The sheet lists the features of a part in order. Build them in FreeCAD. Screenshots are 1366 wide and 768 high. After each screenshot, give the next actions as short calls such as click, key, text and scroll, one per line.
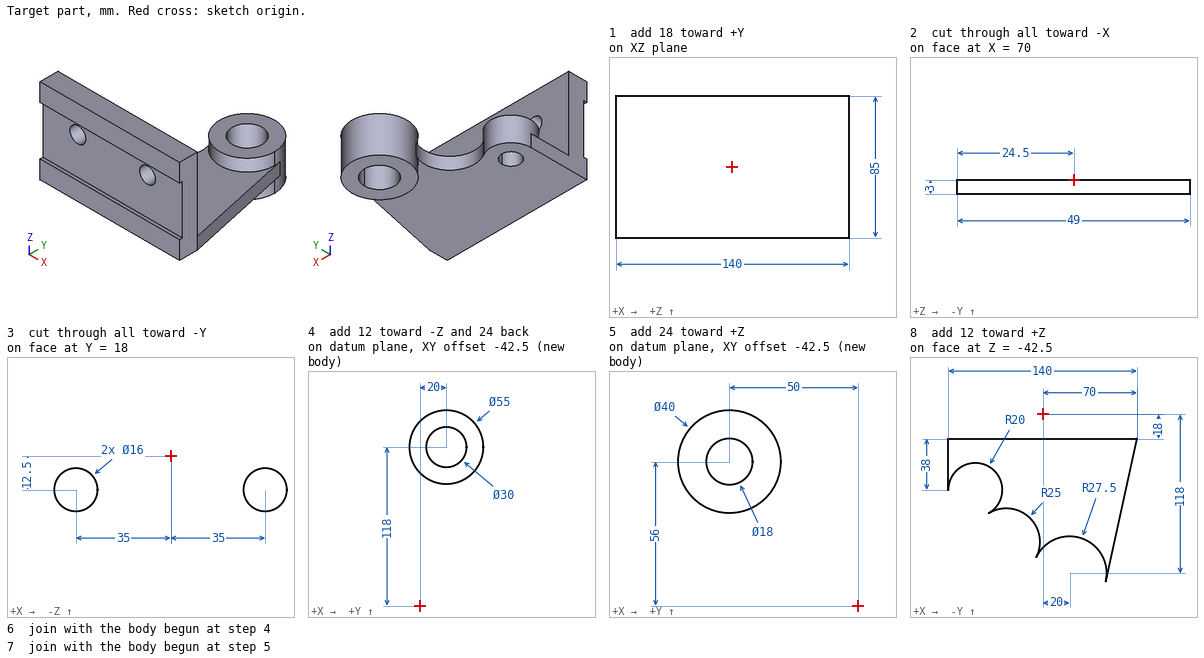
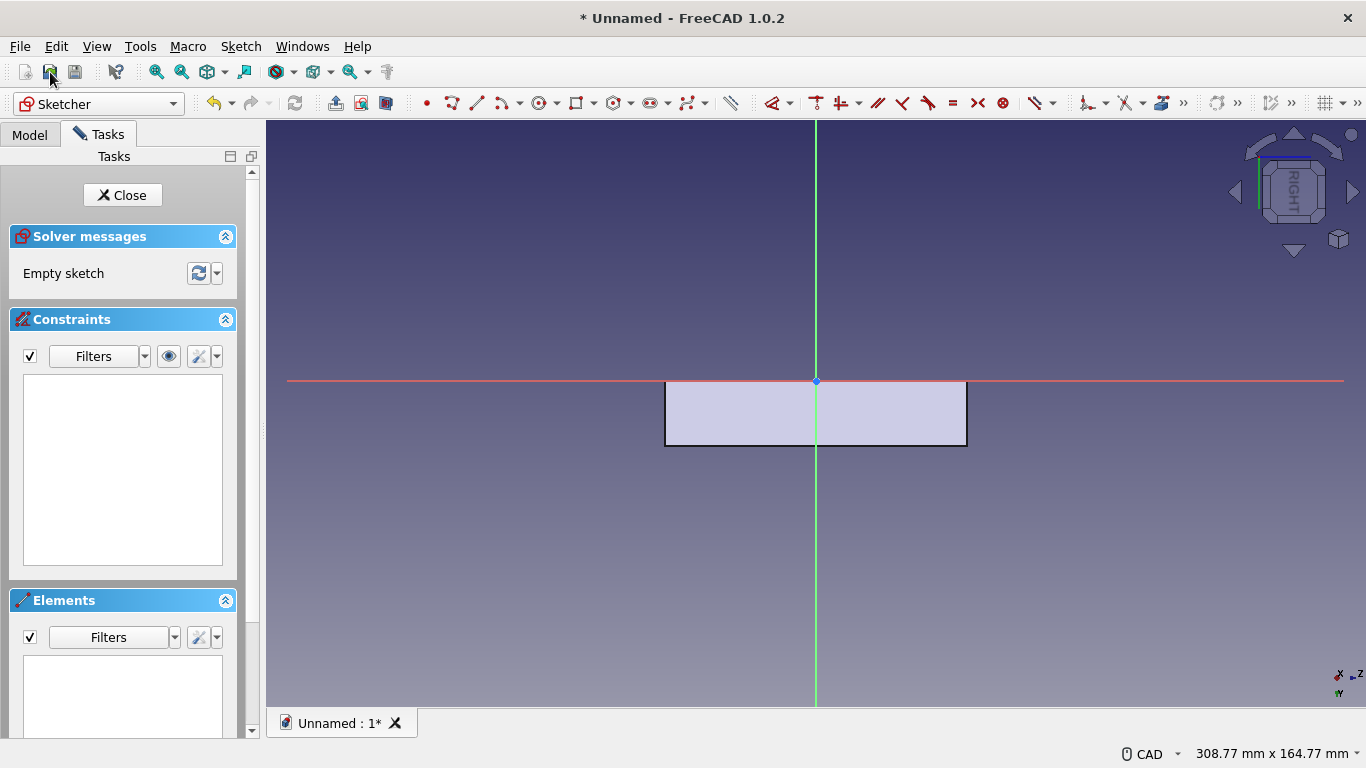
scroll(846, 375, up, 6)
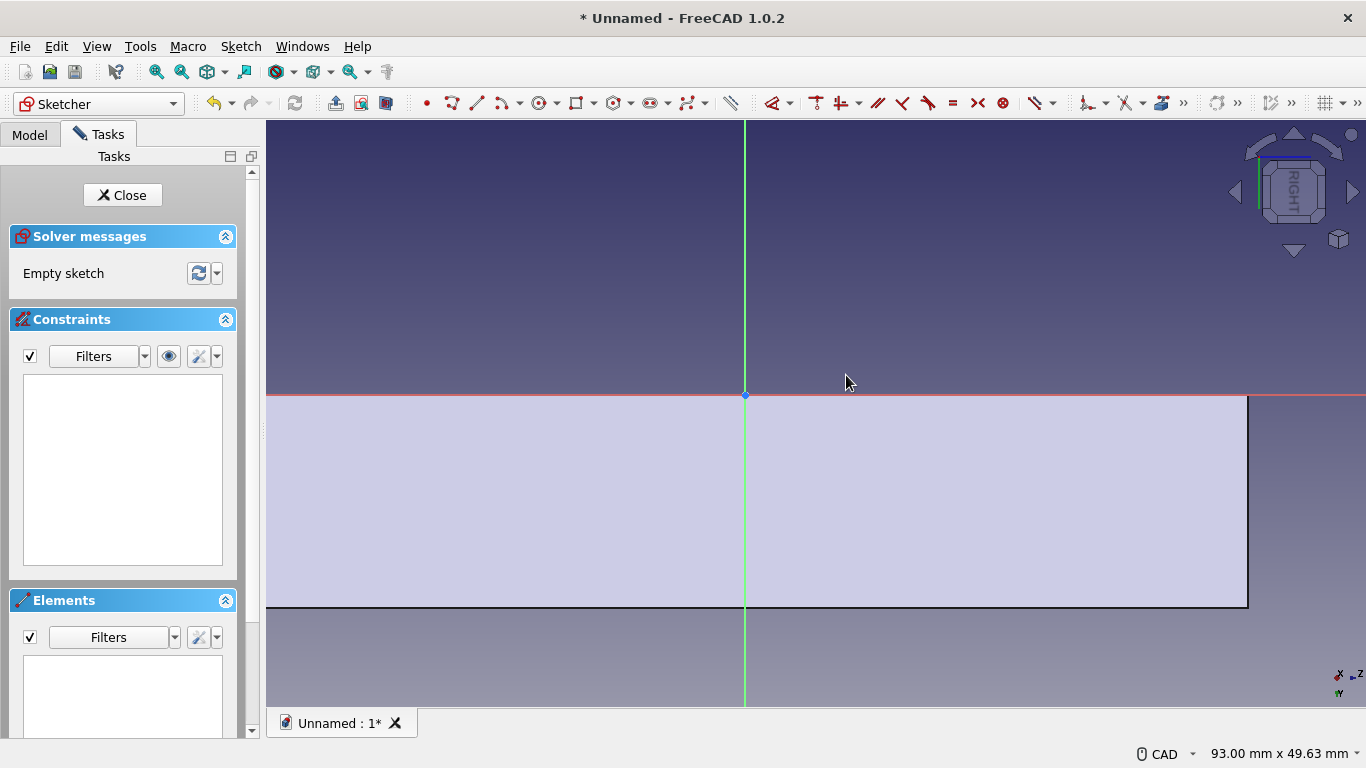
click(576, 104)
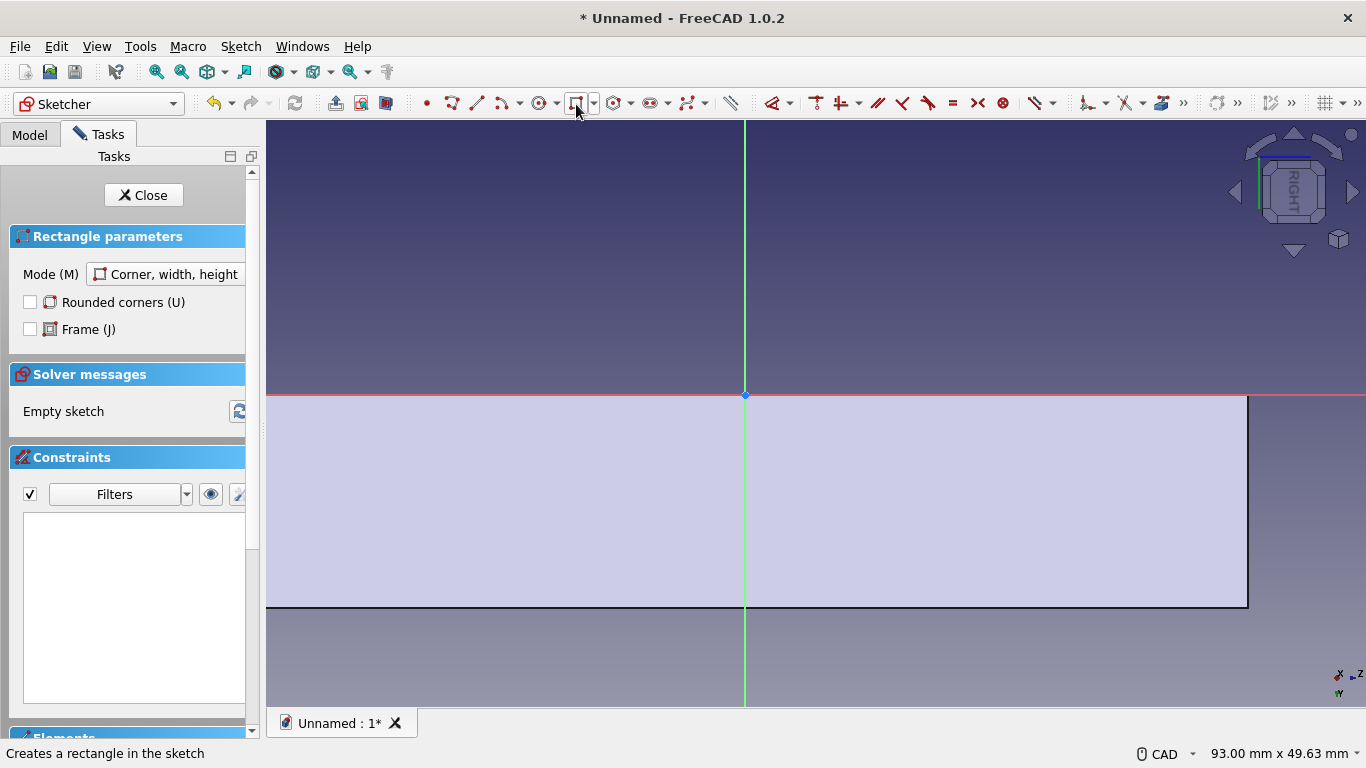
click(455, 395)
click(1035, 431)
key(Escape)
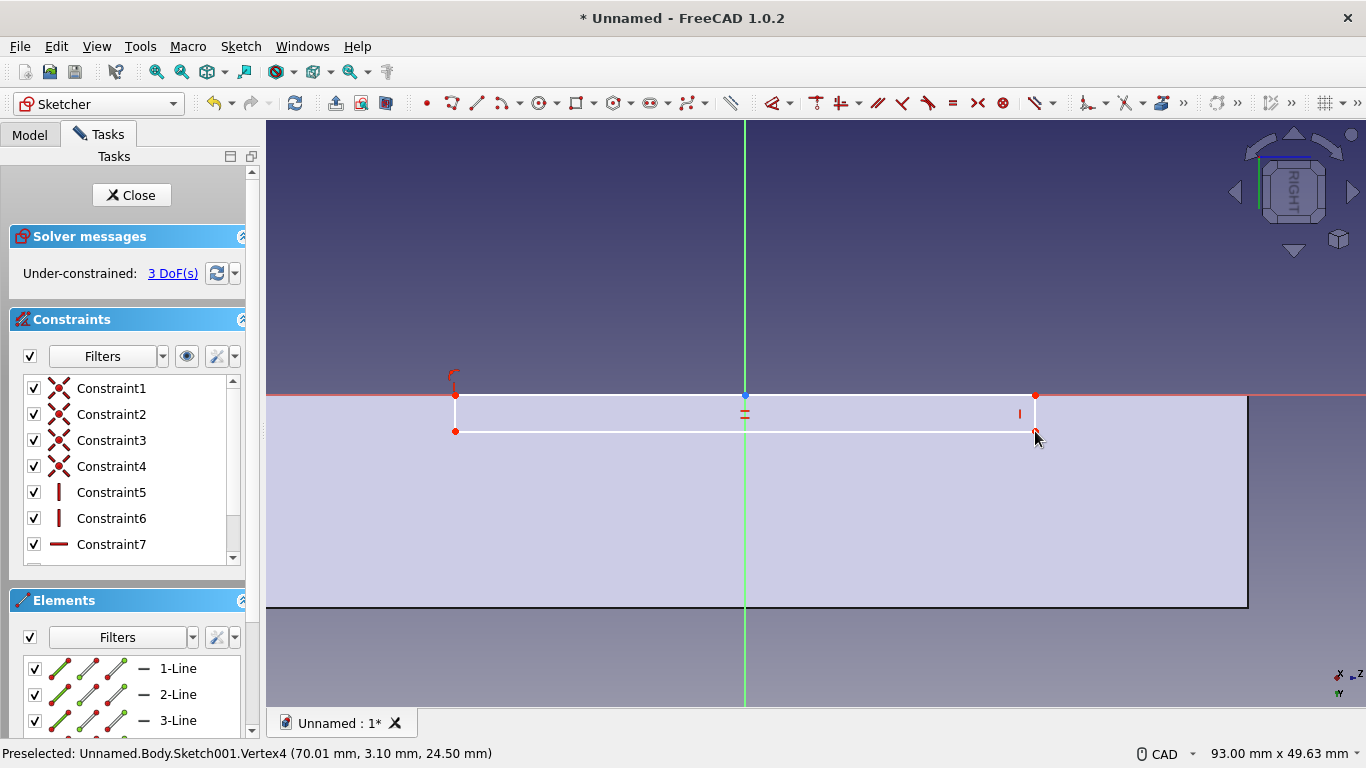
click(772, 104)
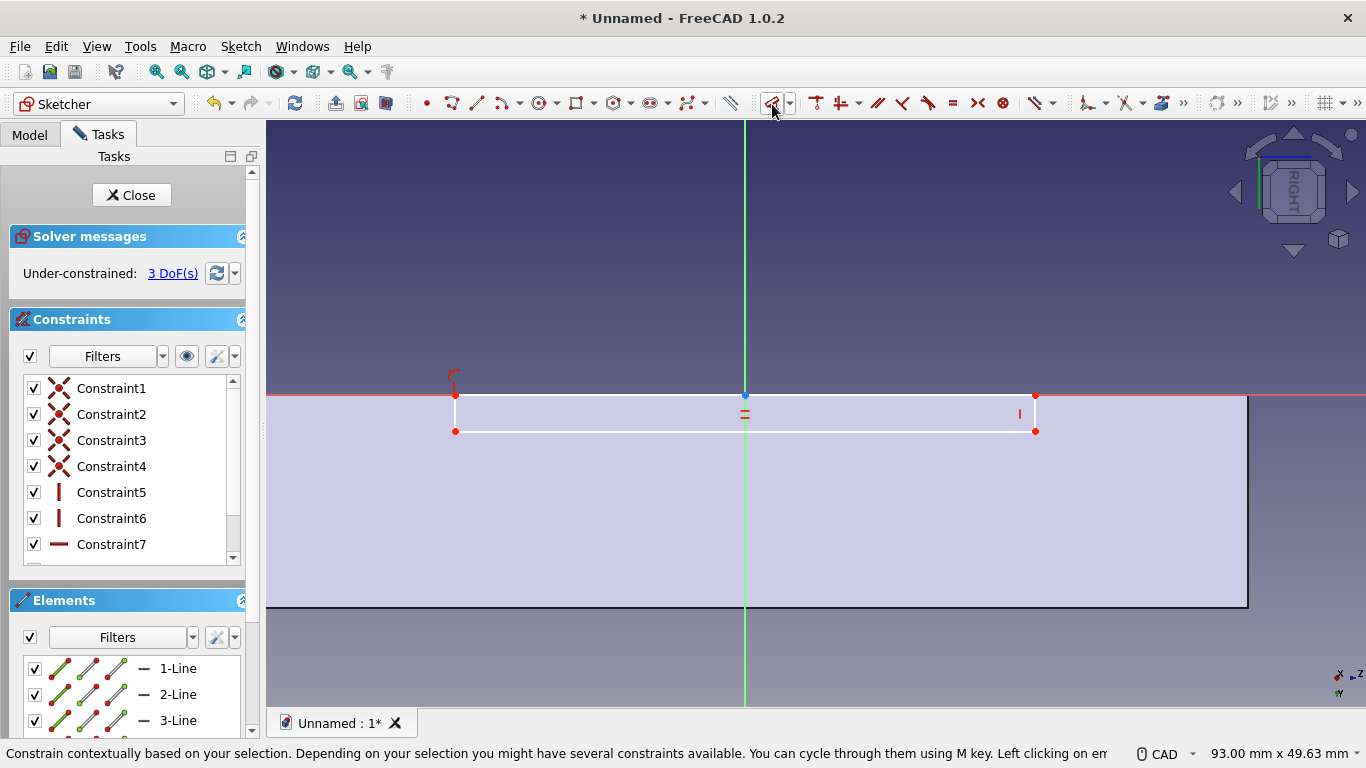
scroll(455, 406, up, 2)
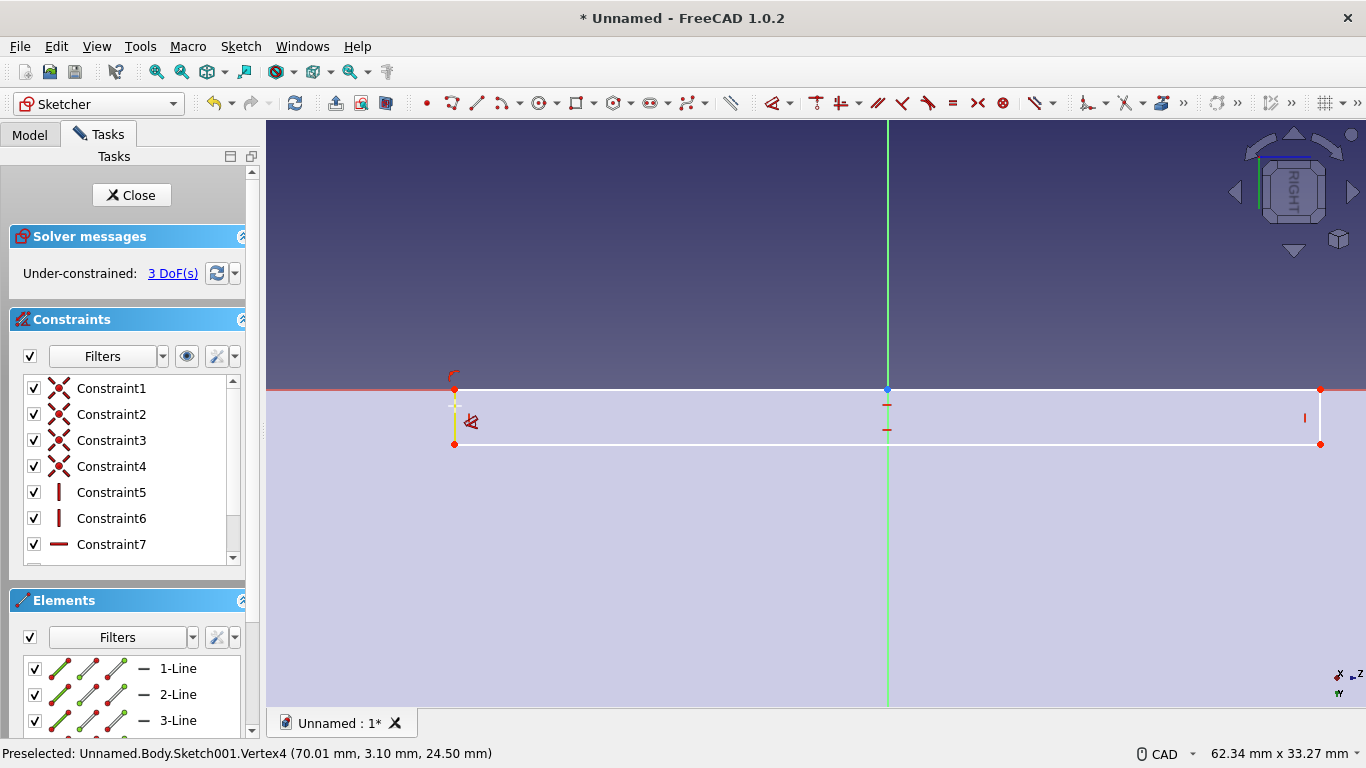
click(455, 406)
click(421, 417)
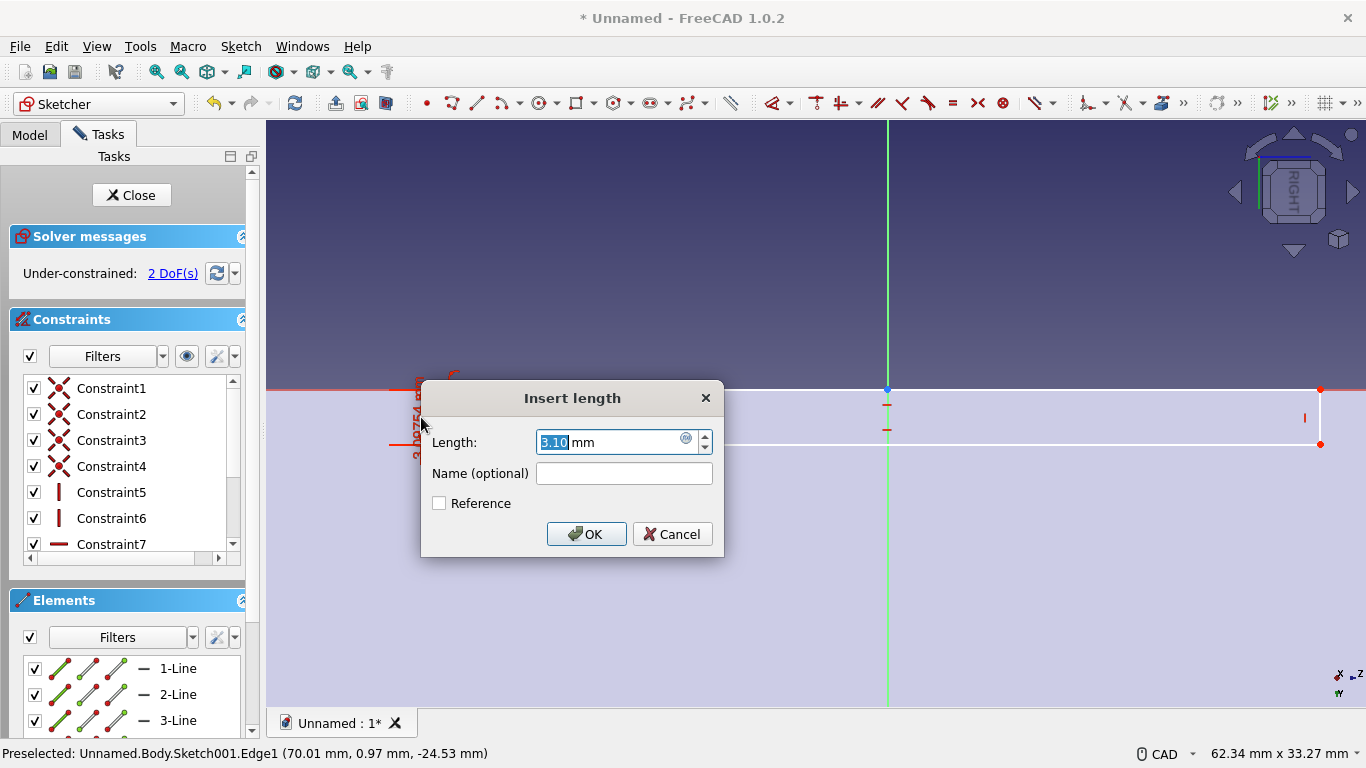
text(3)
key(Return)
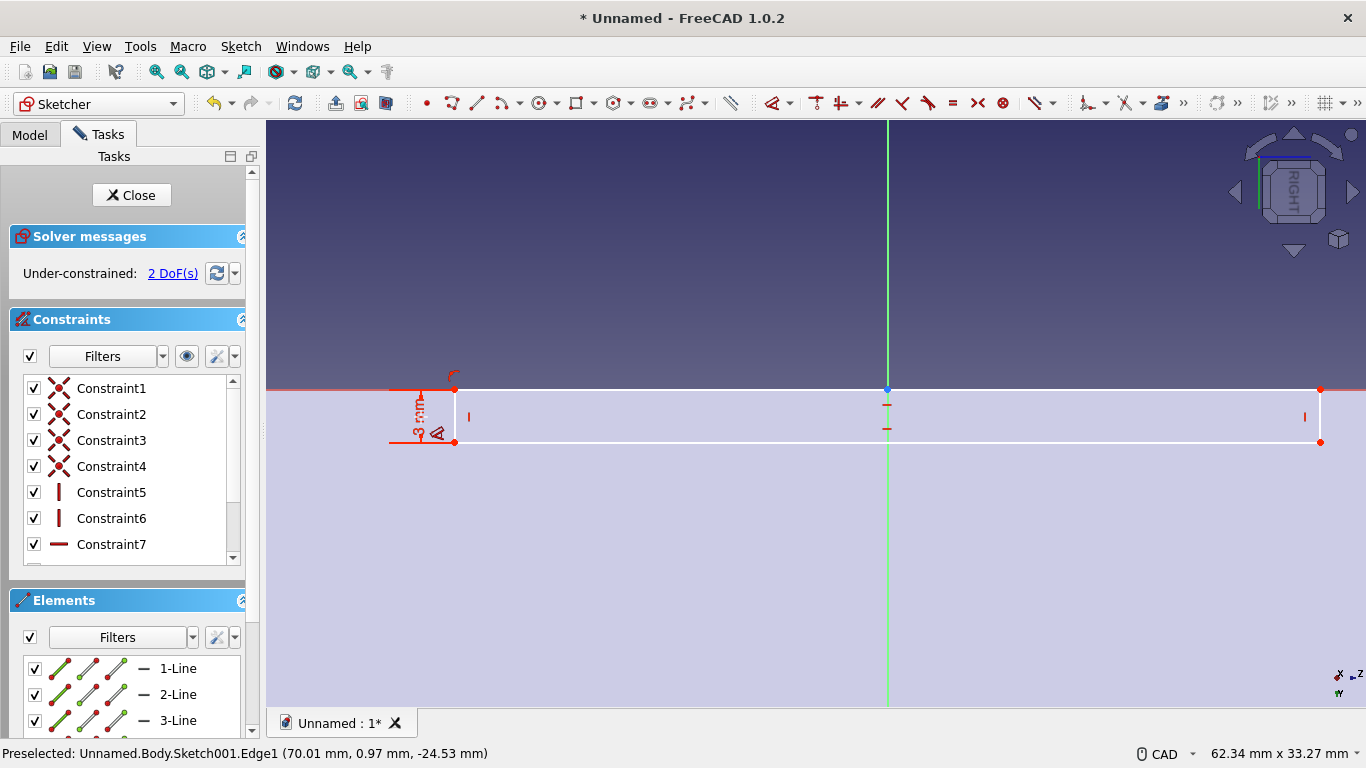
click(714, 443)
click(828, 477)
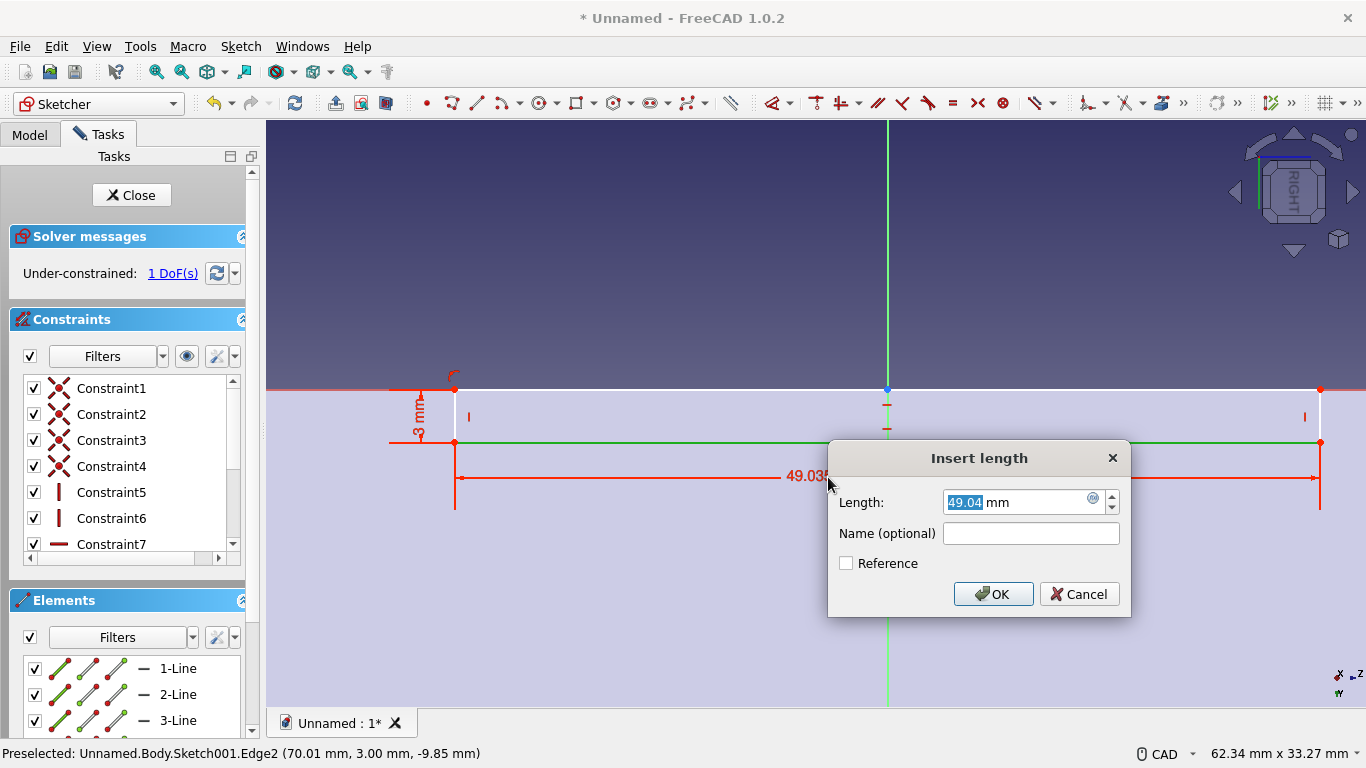
text(49)
key(Return)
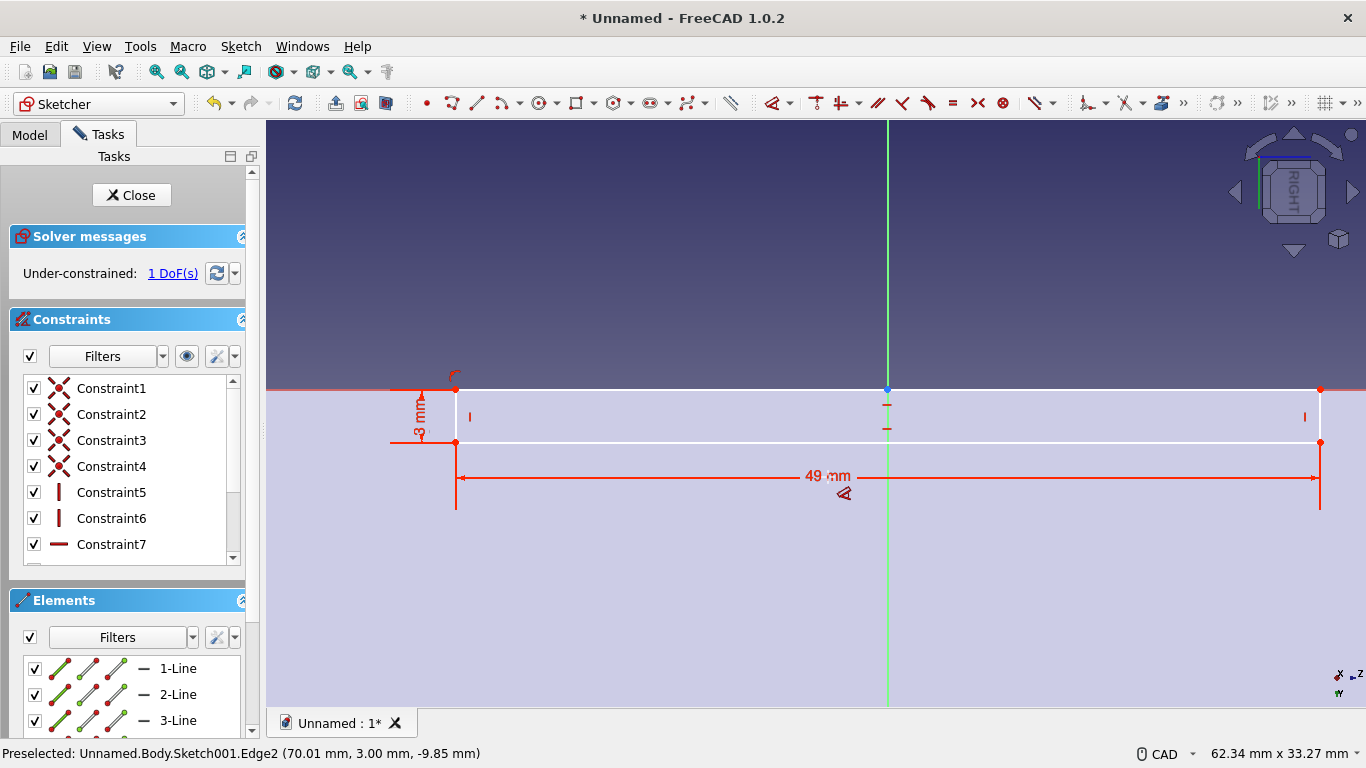
click(456, 390)
click(672, 356)